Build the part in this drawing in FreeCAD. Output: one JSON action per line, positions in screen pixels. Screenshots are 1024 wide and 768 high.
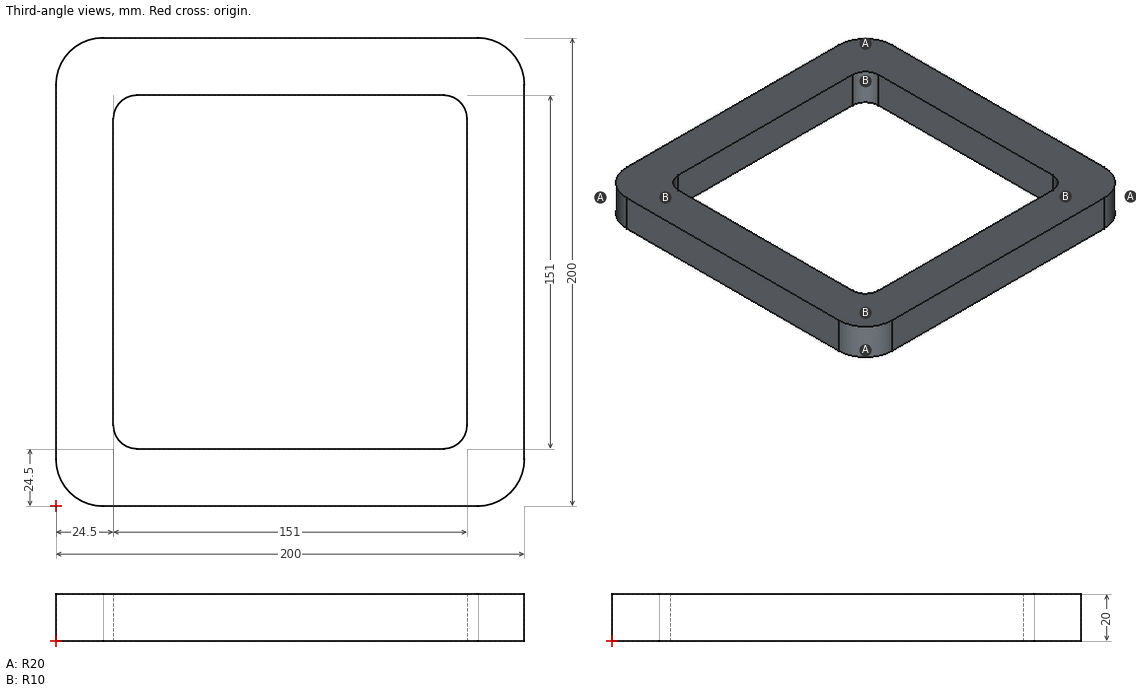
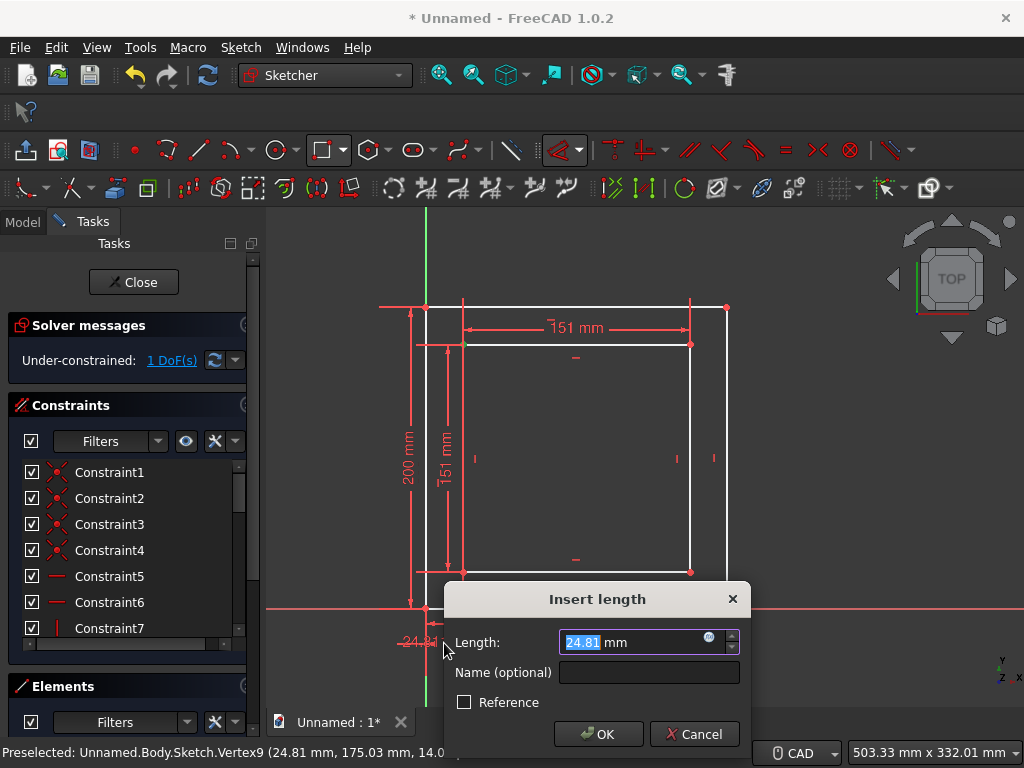
{"action": "type", "text": "24.5"}
{"action": "key", "text": "Return"}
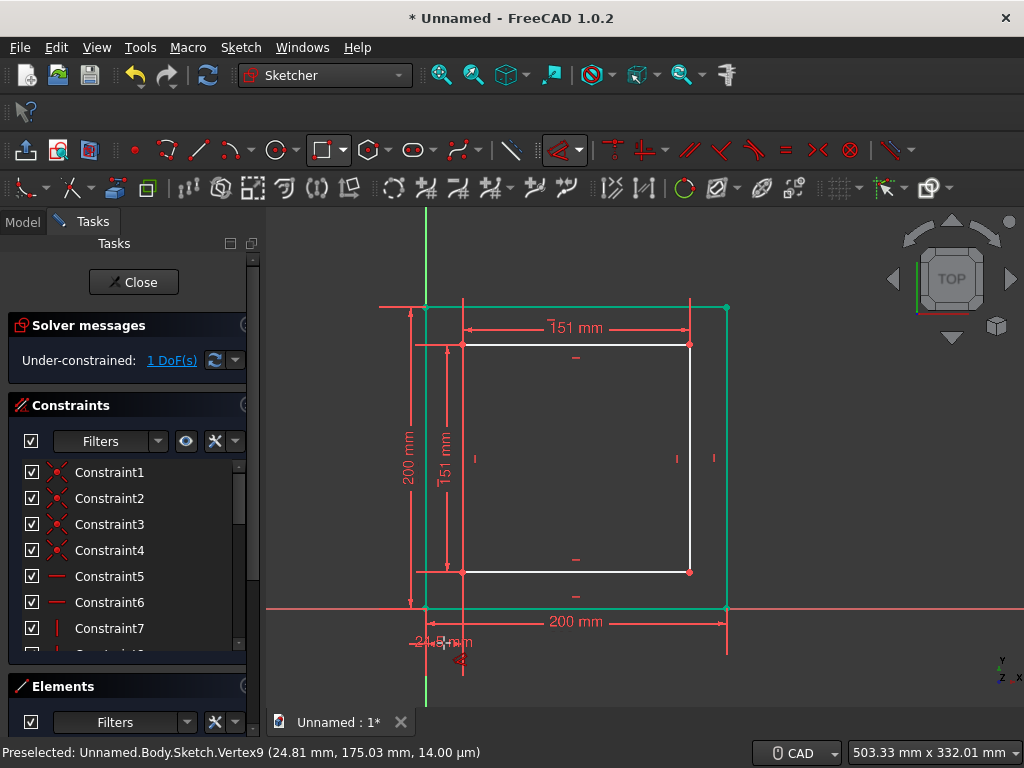
{"action": "left_click", "coordinate": [463, 572]}
{"action": "left_click", "coordinate": [392, 590]}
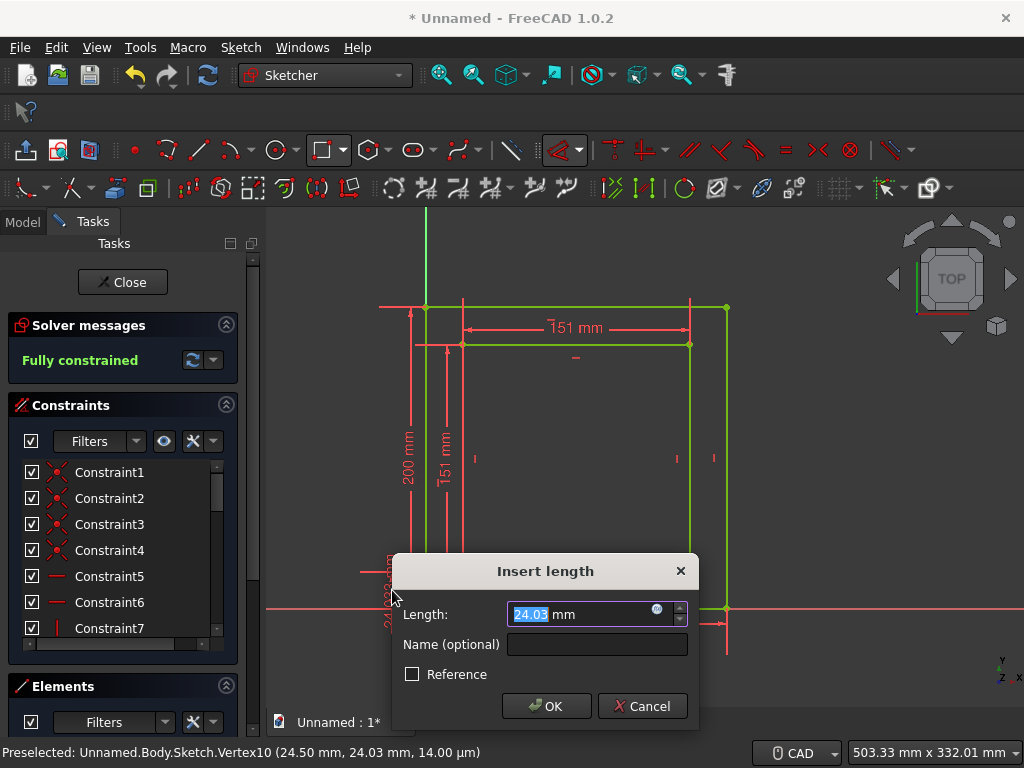
{"action": "type", "text": "24.5"}
{"action": "key", "text": "Return"}
{"action": "key", "text": "Escape"}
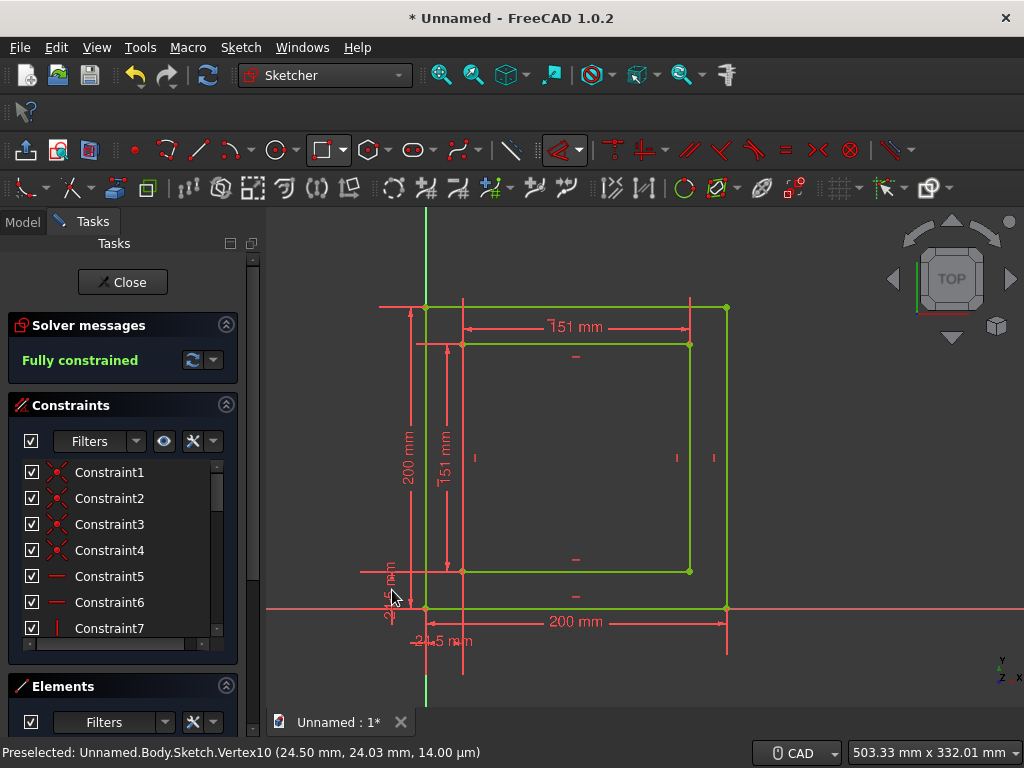
{"action": "left_click", "coordinate": [123, 282]}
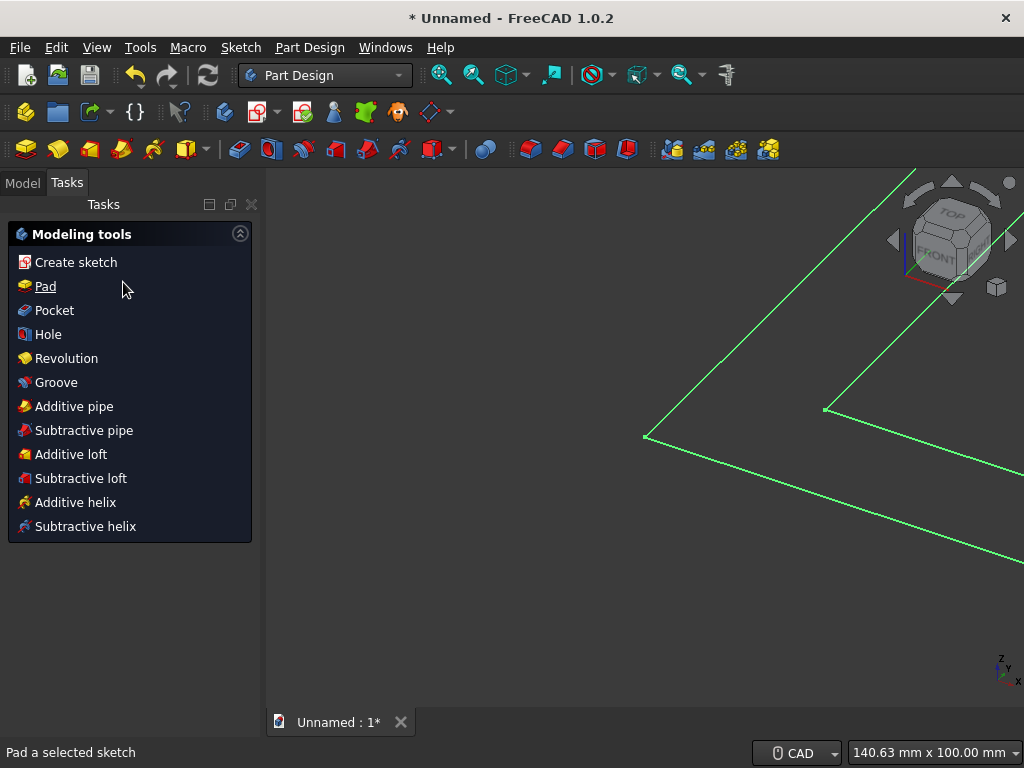
{"action": "left_click", "coordinate": [26, 150]}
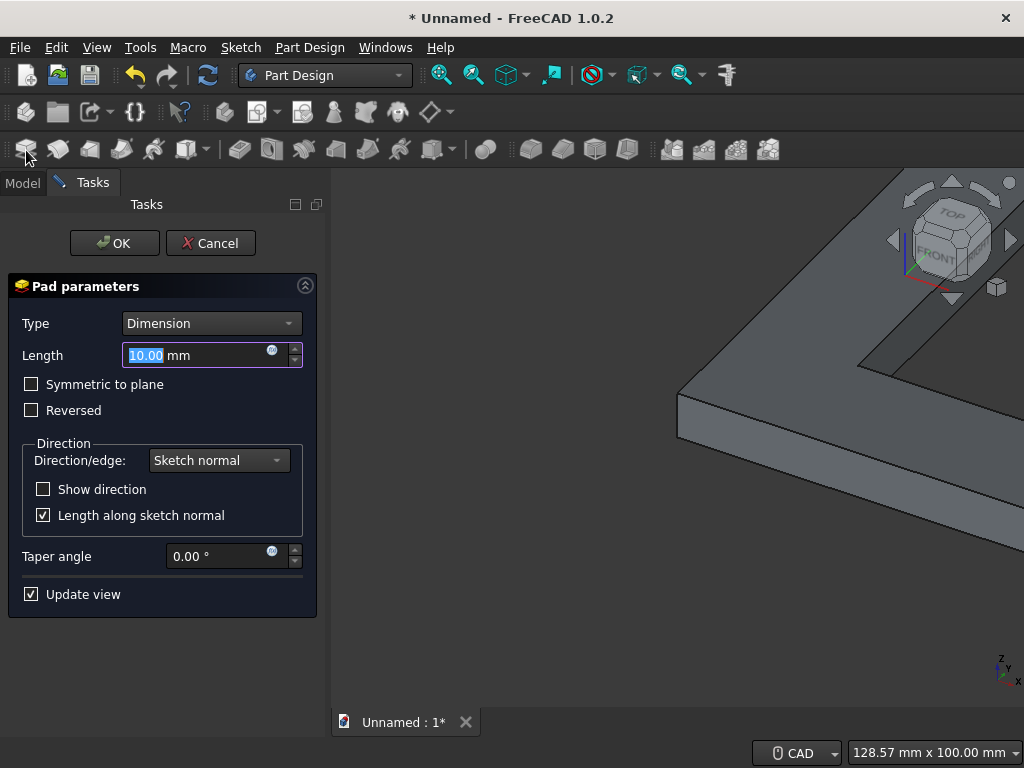
{"action": "type", "text": "20"}
{"action": "key", "text": "Tab"}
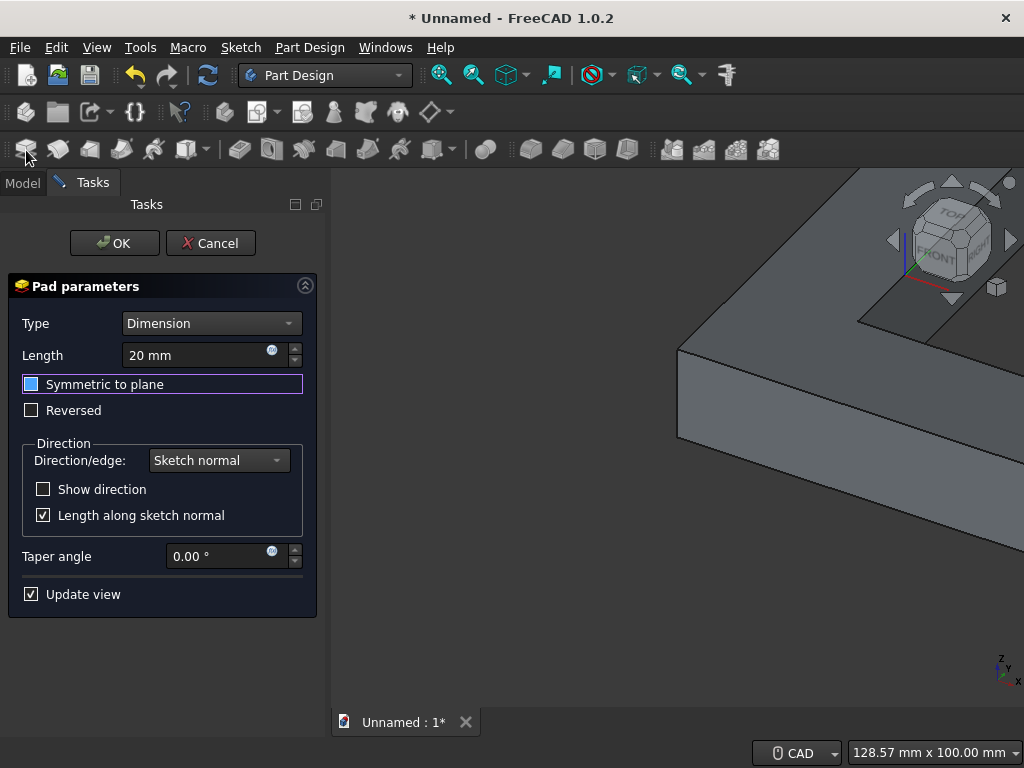
{"action": "left_click", "coordinate": [115, 243]}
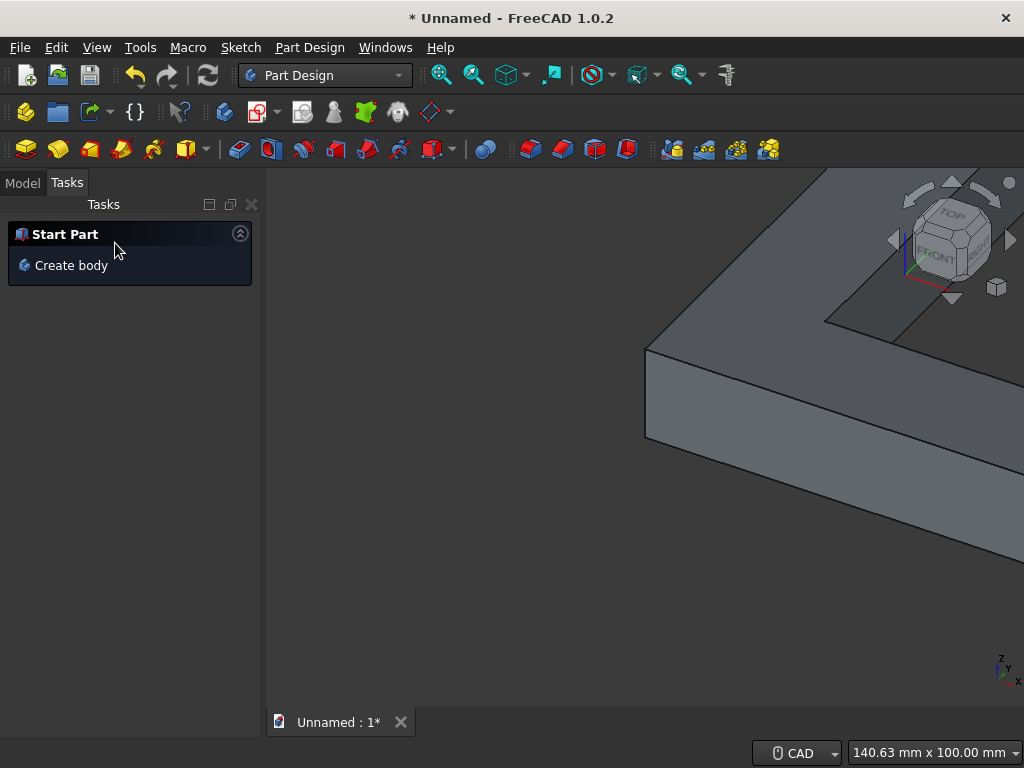
{"action": "left_click", "coordinate": [442, 76]}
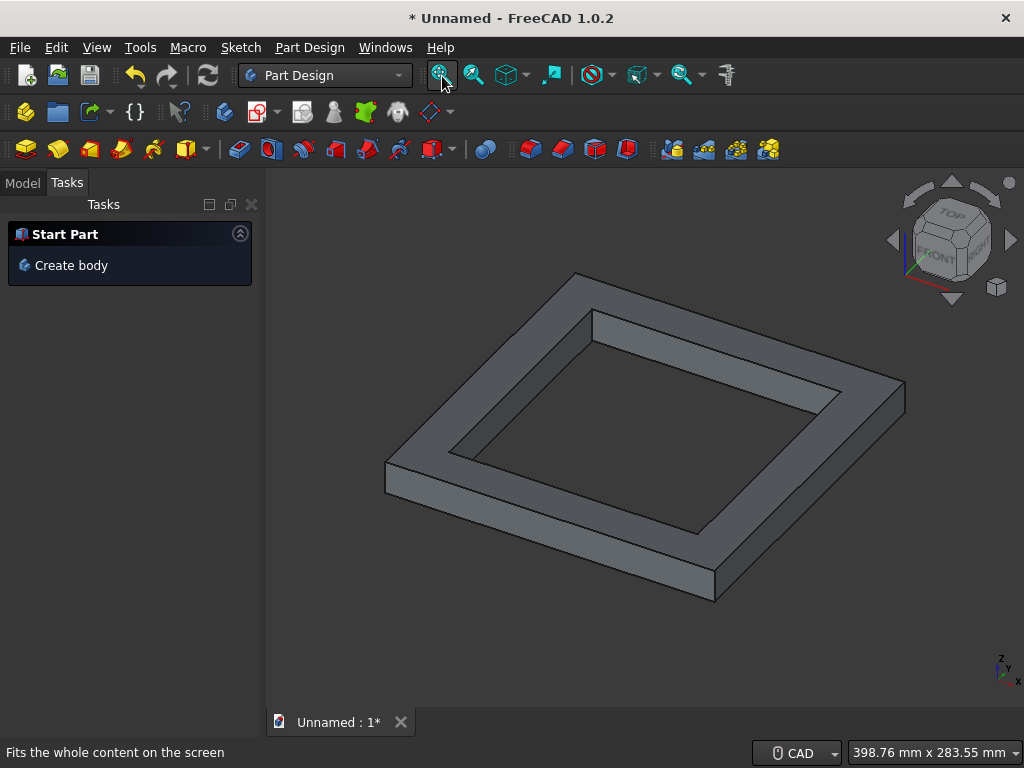
{"action": "left_click", "coordinate": [715, 585]}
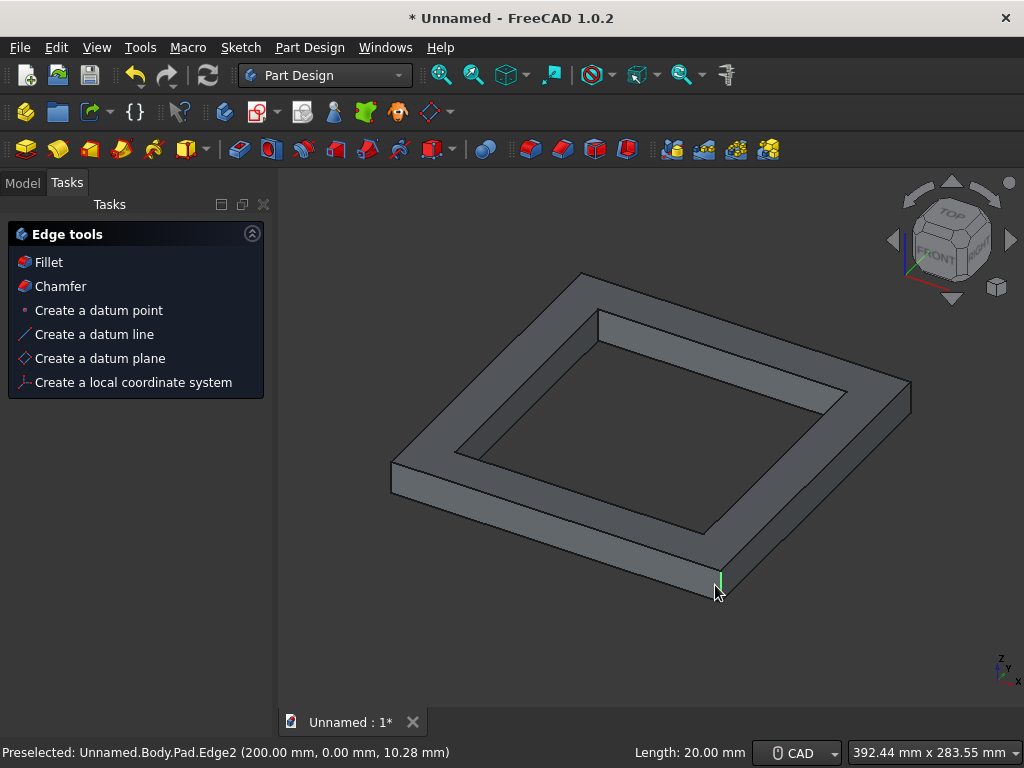
{"action": "key", "text": "0"}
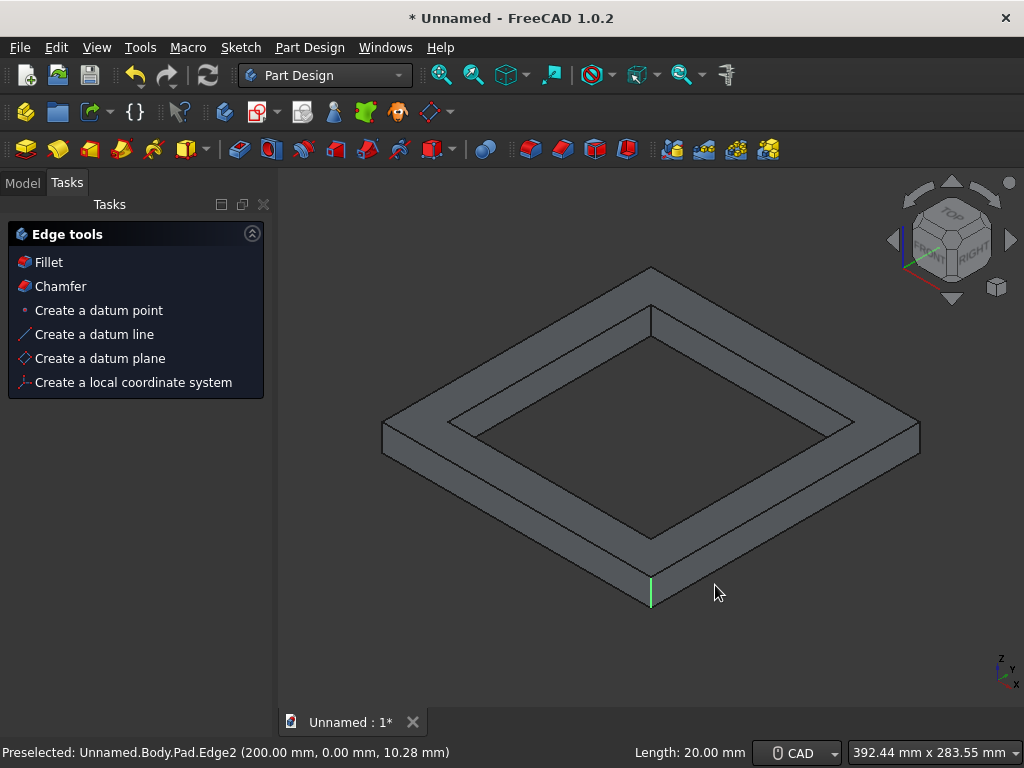
{"action": "key", "text": "2"}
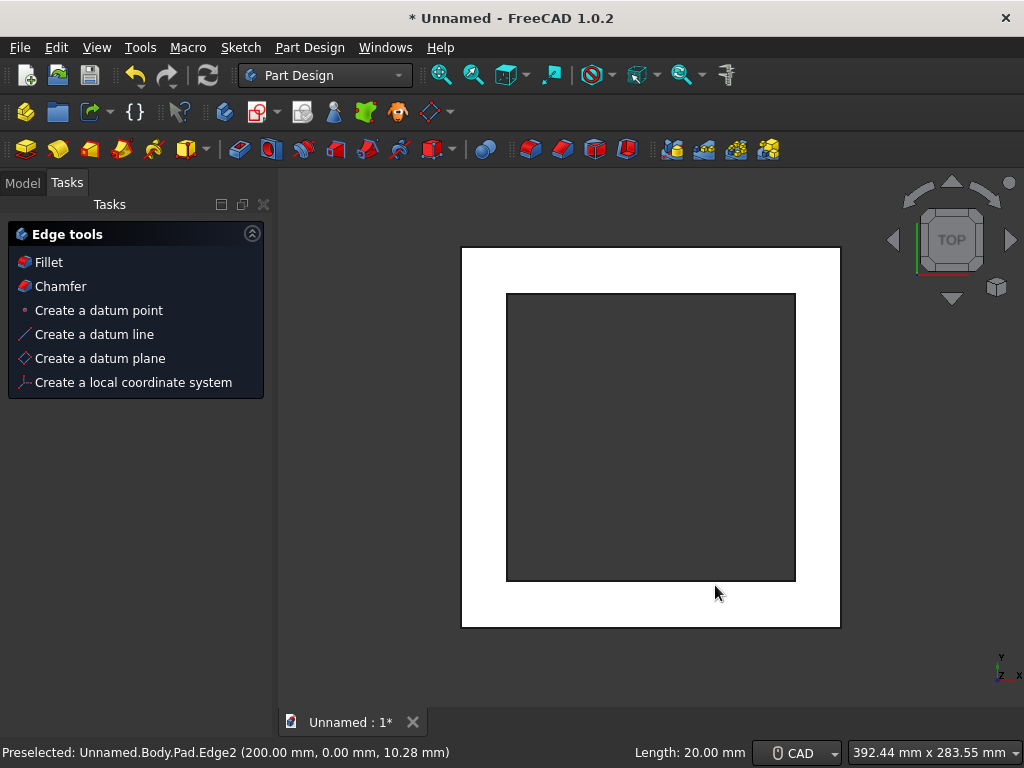
{"action": "key", "text": "1"}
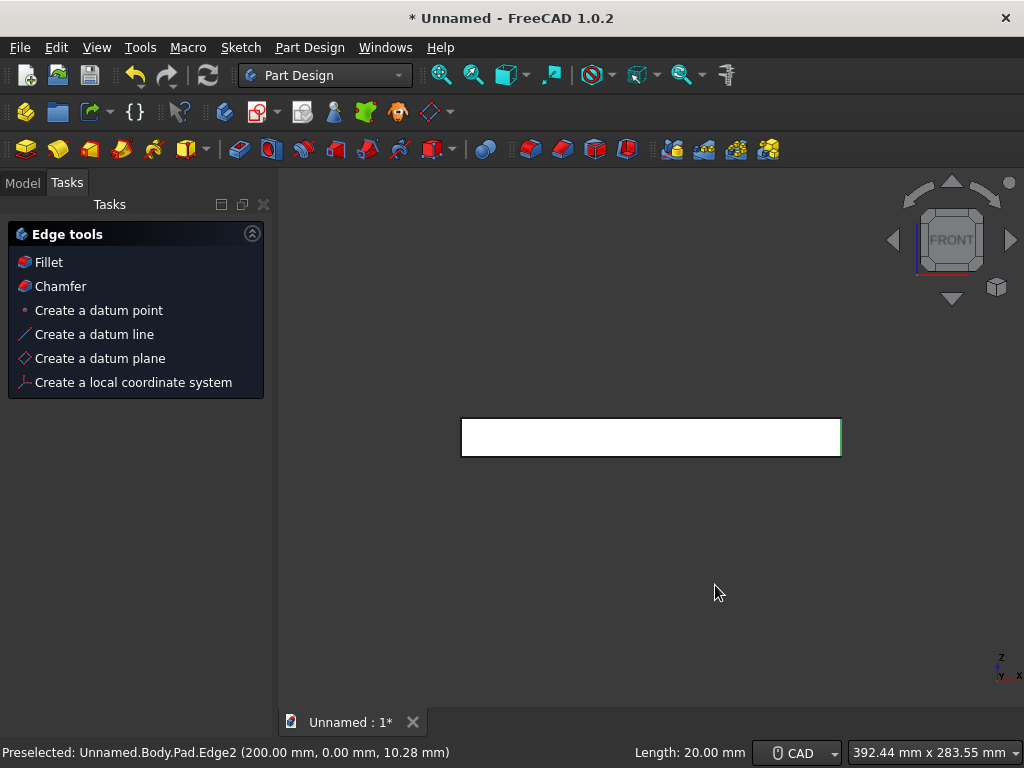
{"action": "left_click", "coordinate": [461, 436], "text": "ctrl"}